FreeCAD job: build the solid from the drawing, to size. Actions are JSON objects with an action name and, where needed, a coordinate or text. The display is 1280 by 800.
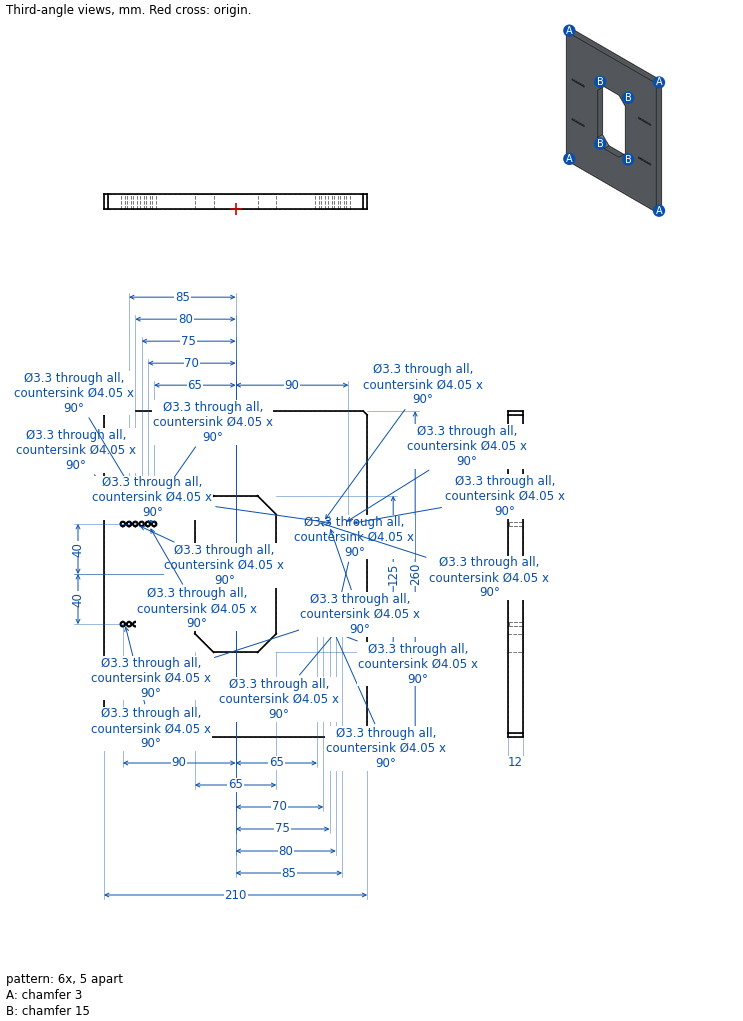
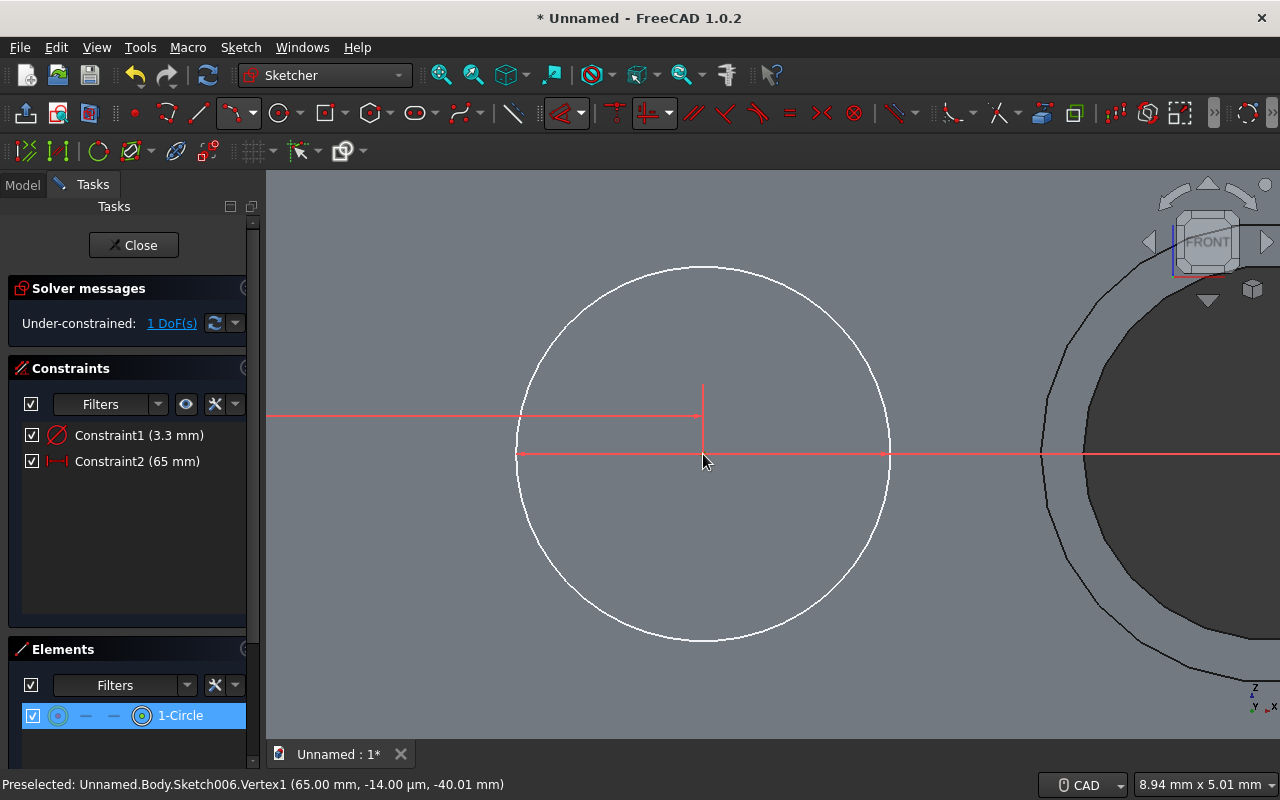
{"action": "left_click", "coordinate": [584, 114]}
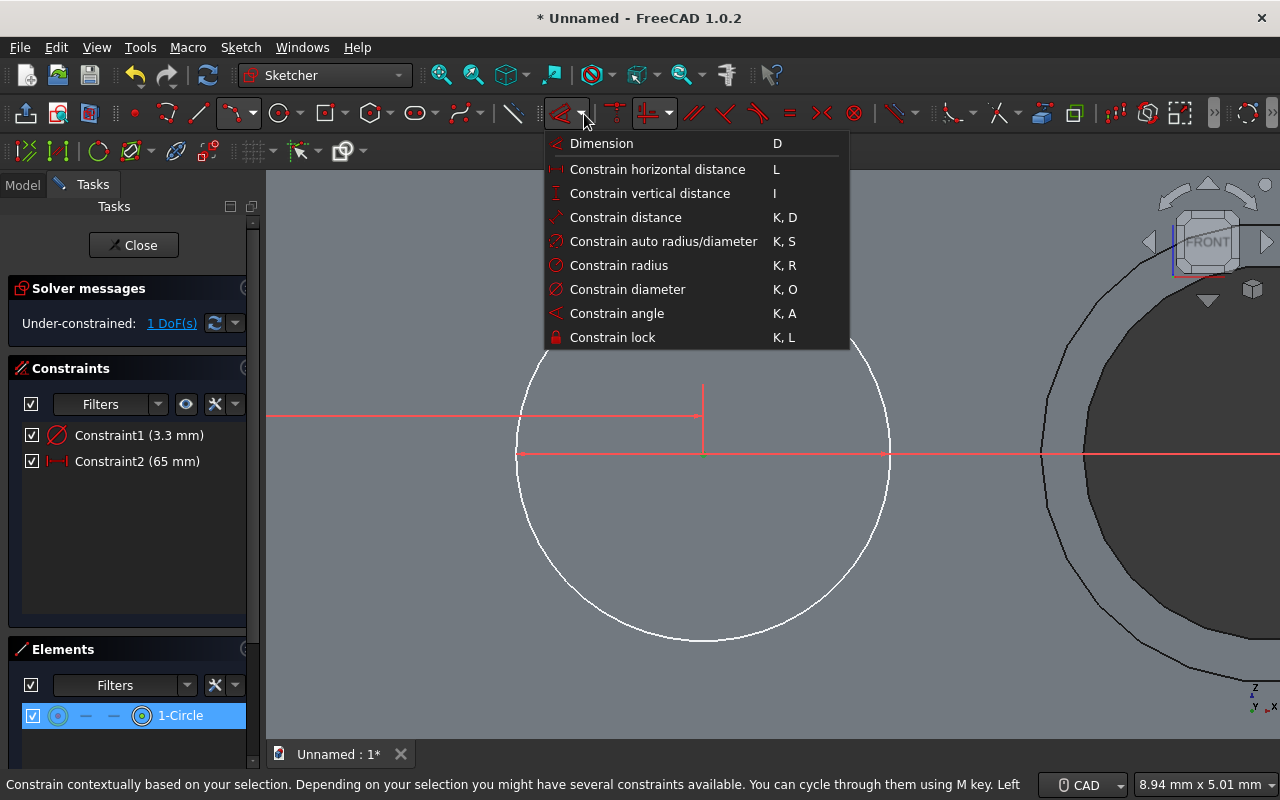
{"action": "left_click", "coordinate": [697, 193]}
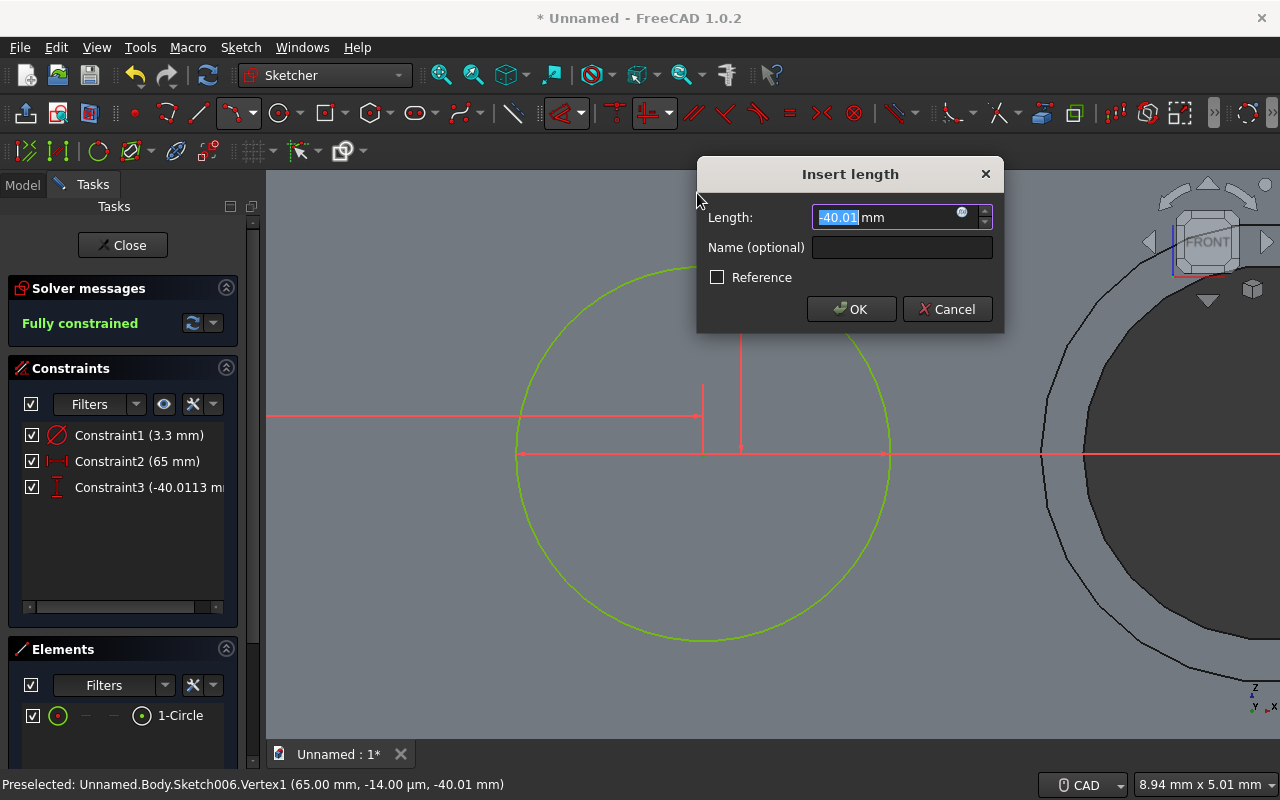
{"action": "type", "text": "-40"}
{"action": "key", "text": "Return"}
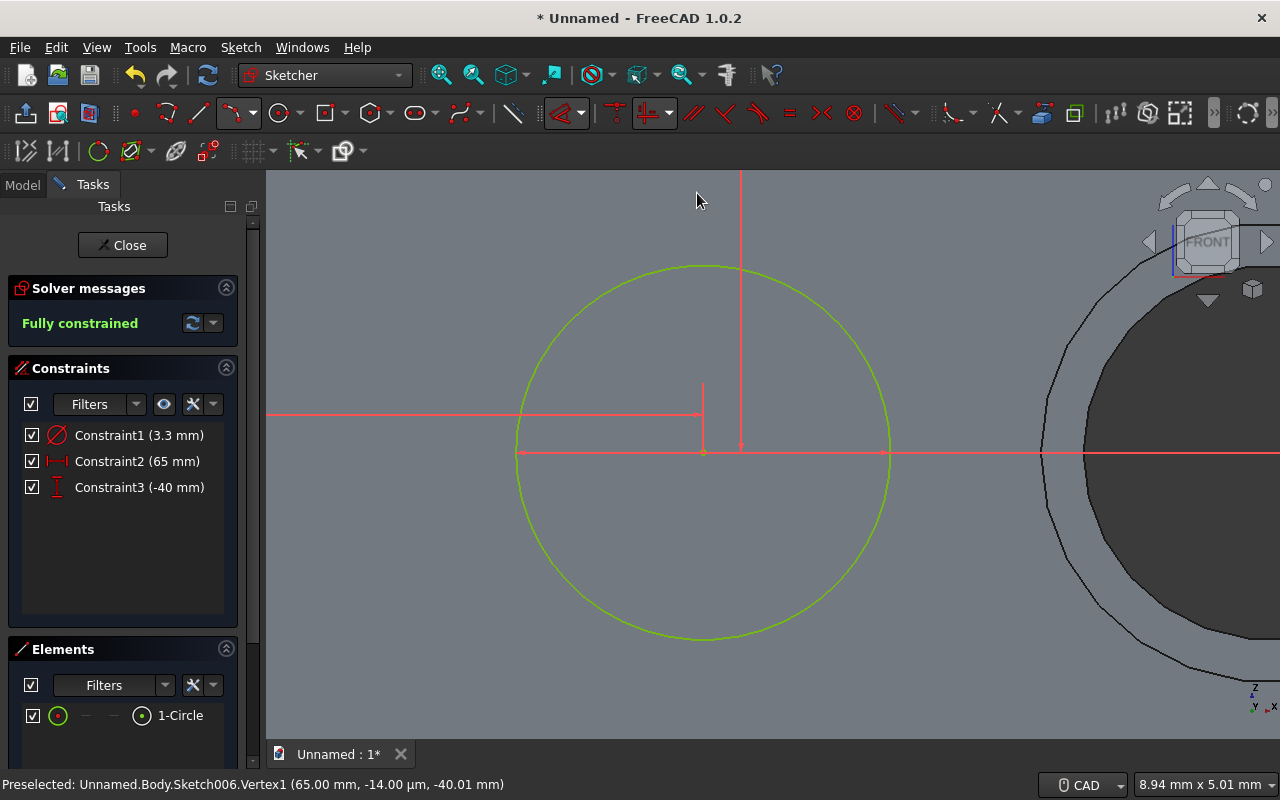
{"action": "left_click", "coordinate": [123, 245]}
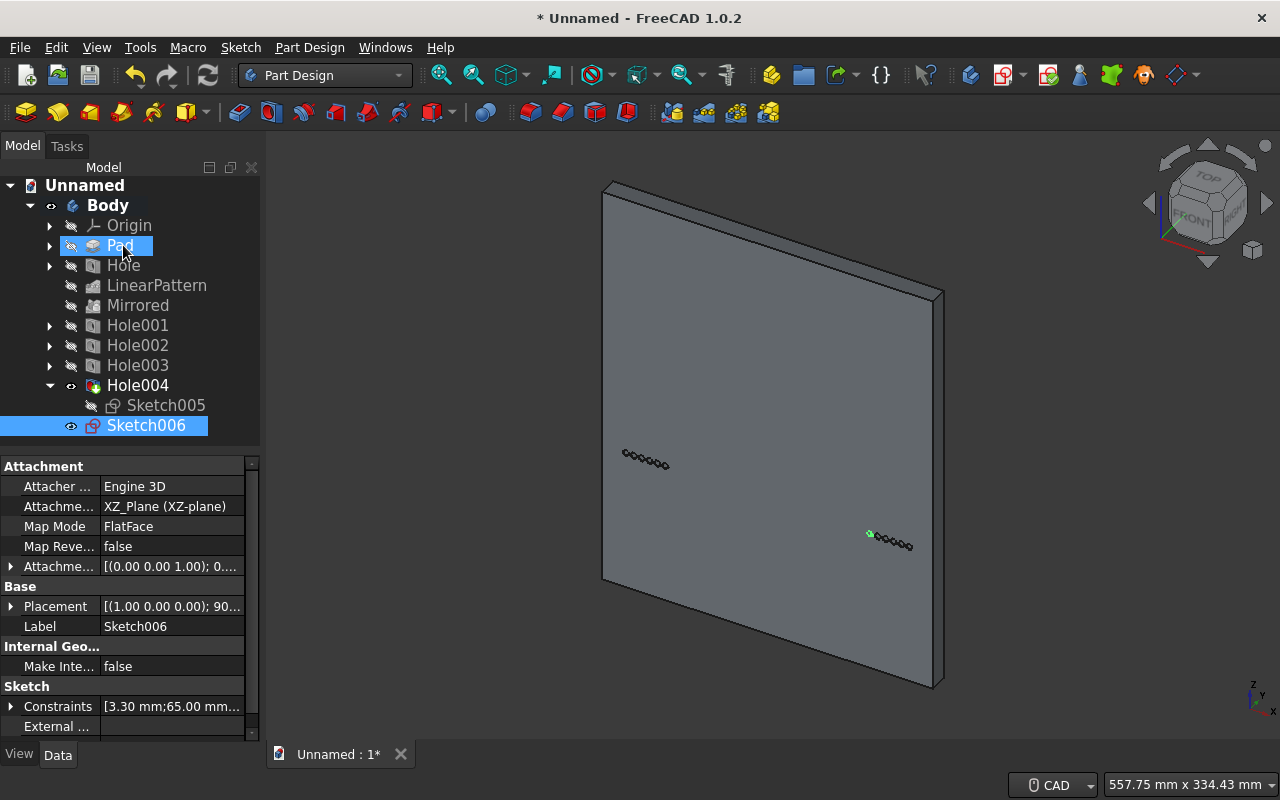
{"action": "left_click", "coordinate": [272, 112]}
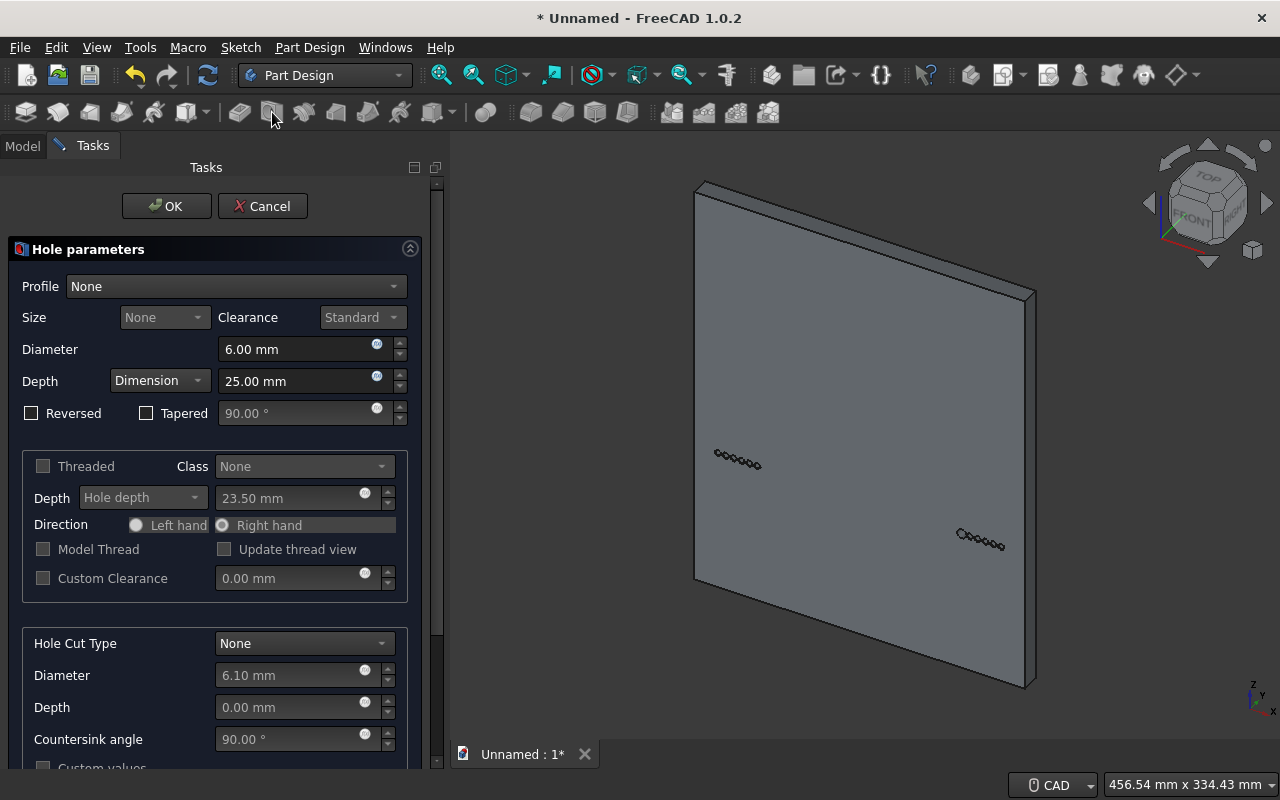
{"action": "triple_click", "coordinate": [305, 349]}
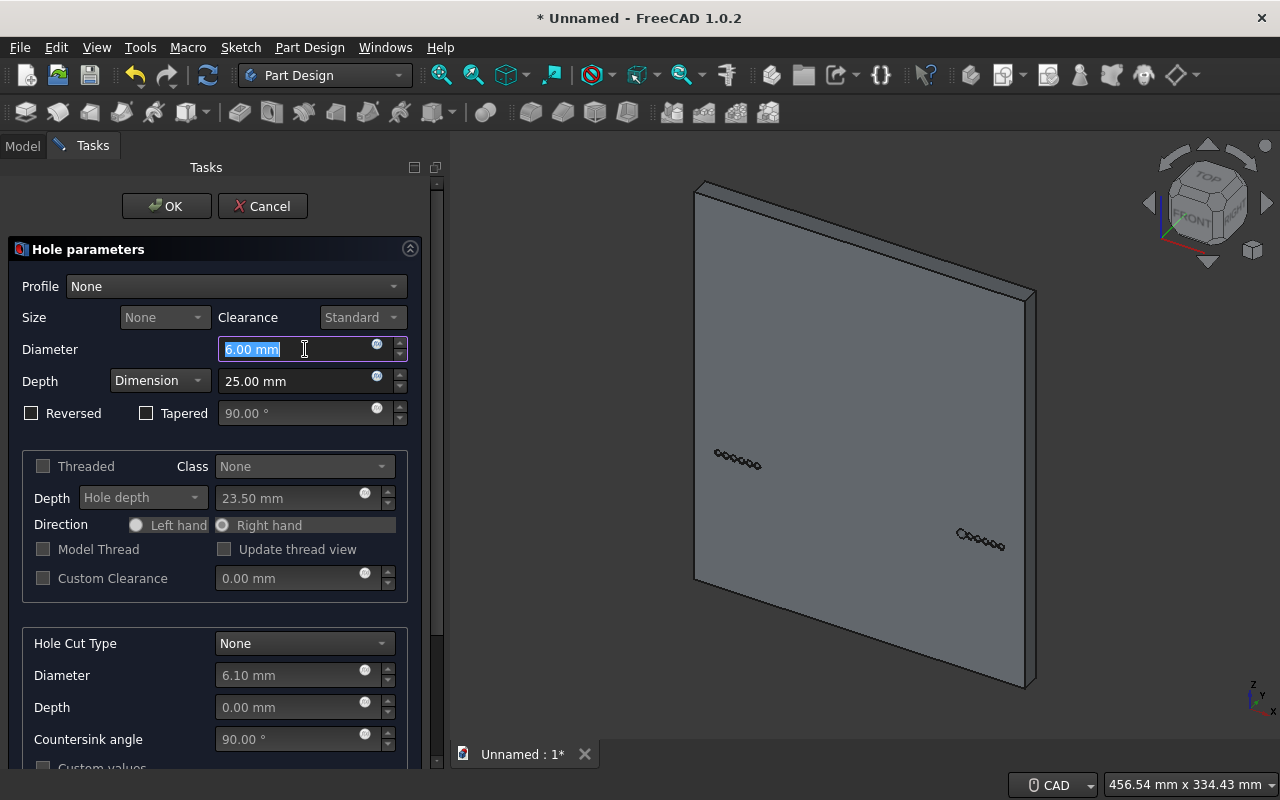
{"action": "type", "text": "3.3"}
{"action": "key", "text": "Tab"}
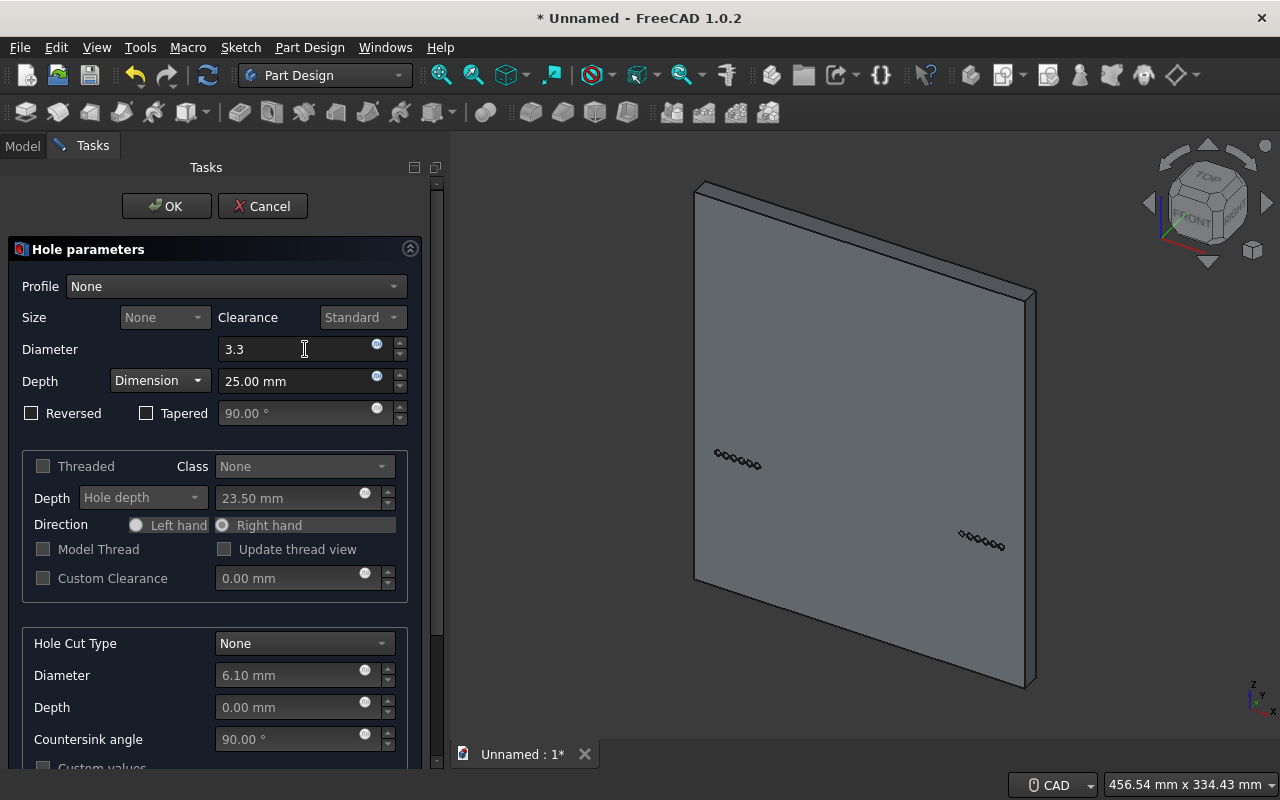
{"action": "left_click", "coordinate": [161, 380]}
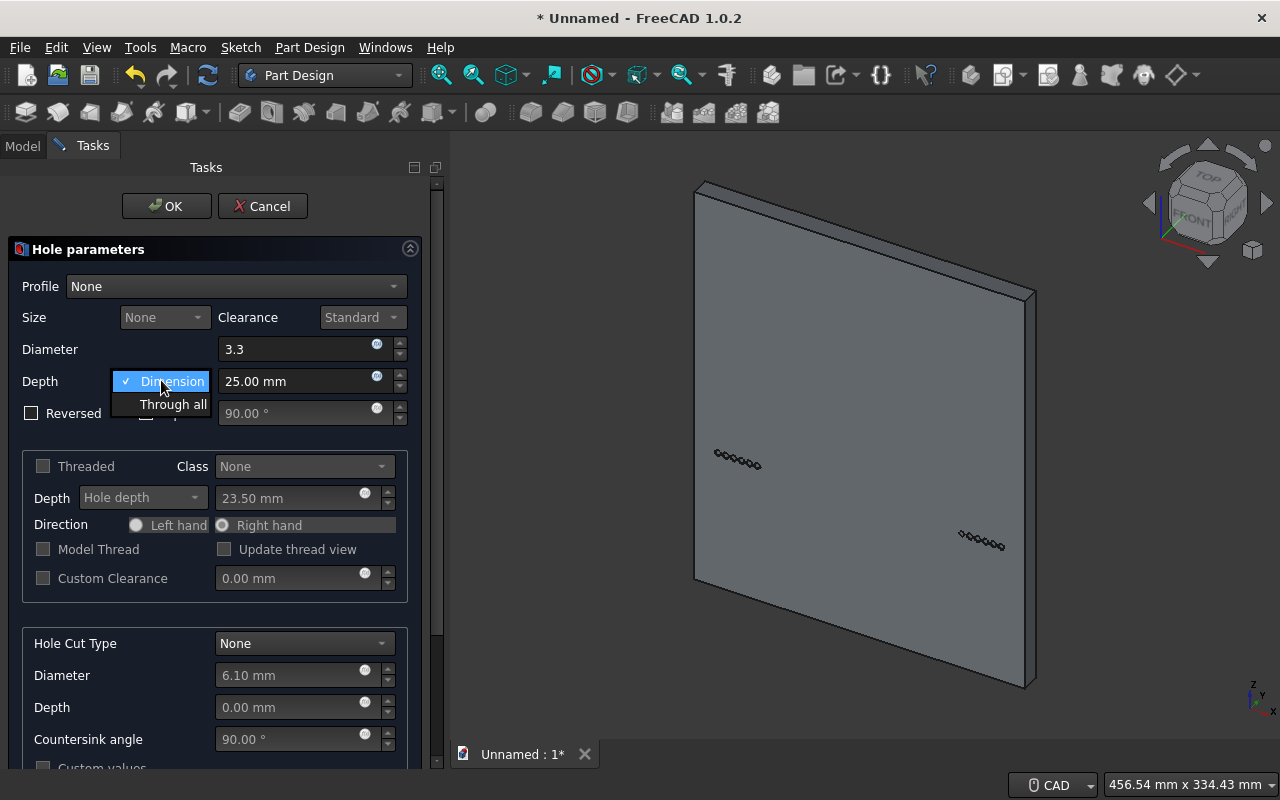
{"action": "left_click", "coordinate": [160, 404]}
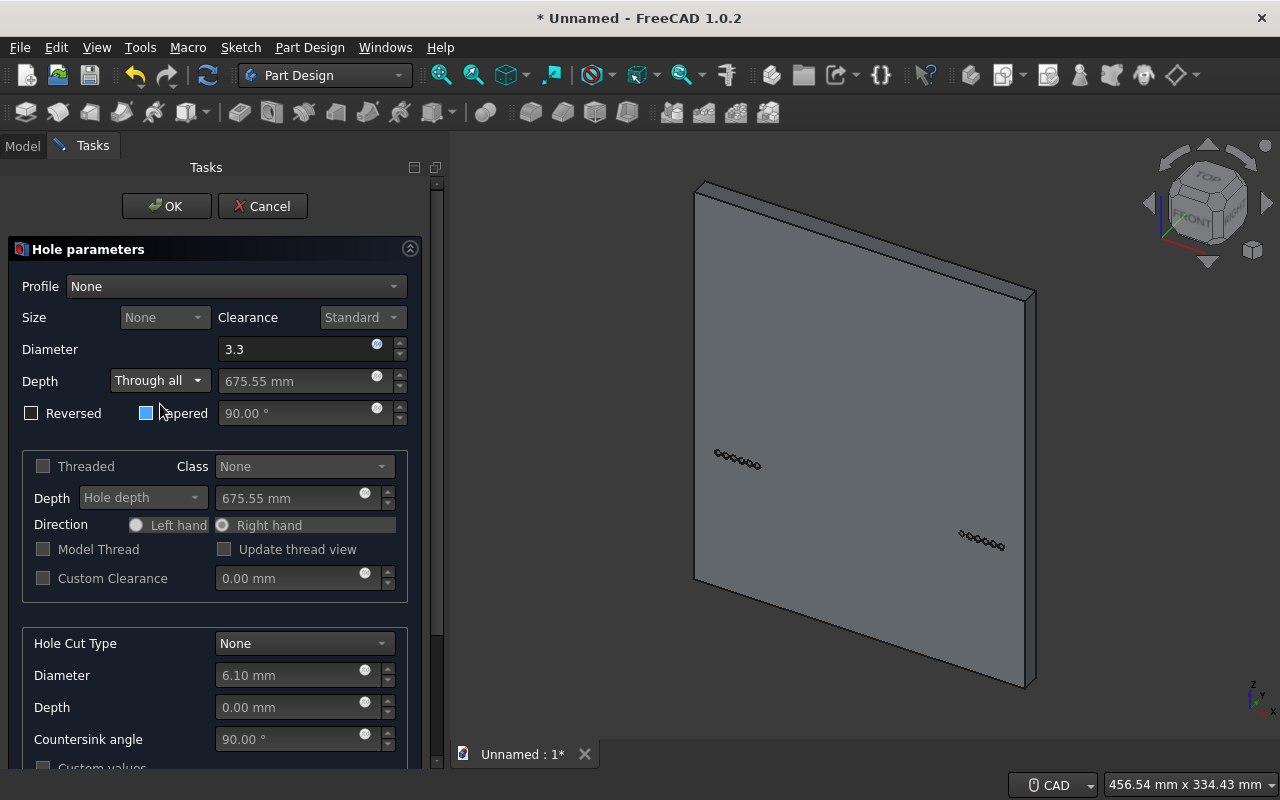
{"action": "left_click", "coordinate": [306, 644]}